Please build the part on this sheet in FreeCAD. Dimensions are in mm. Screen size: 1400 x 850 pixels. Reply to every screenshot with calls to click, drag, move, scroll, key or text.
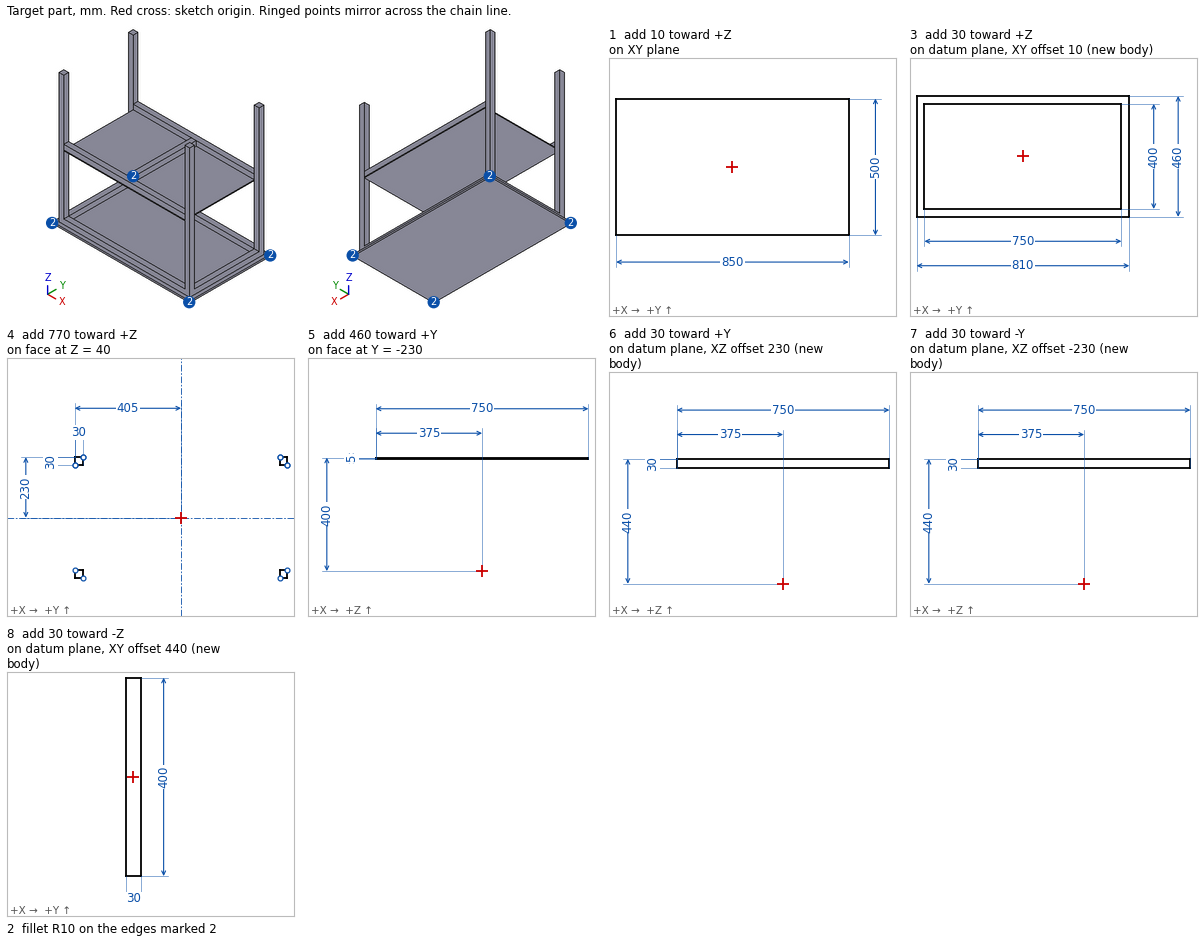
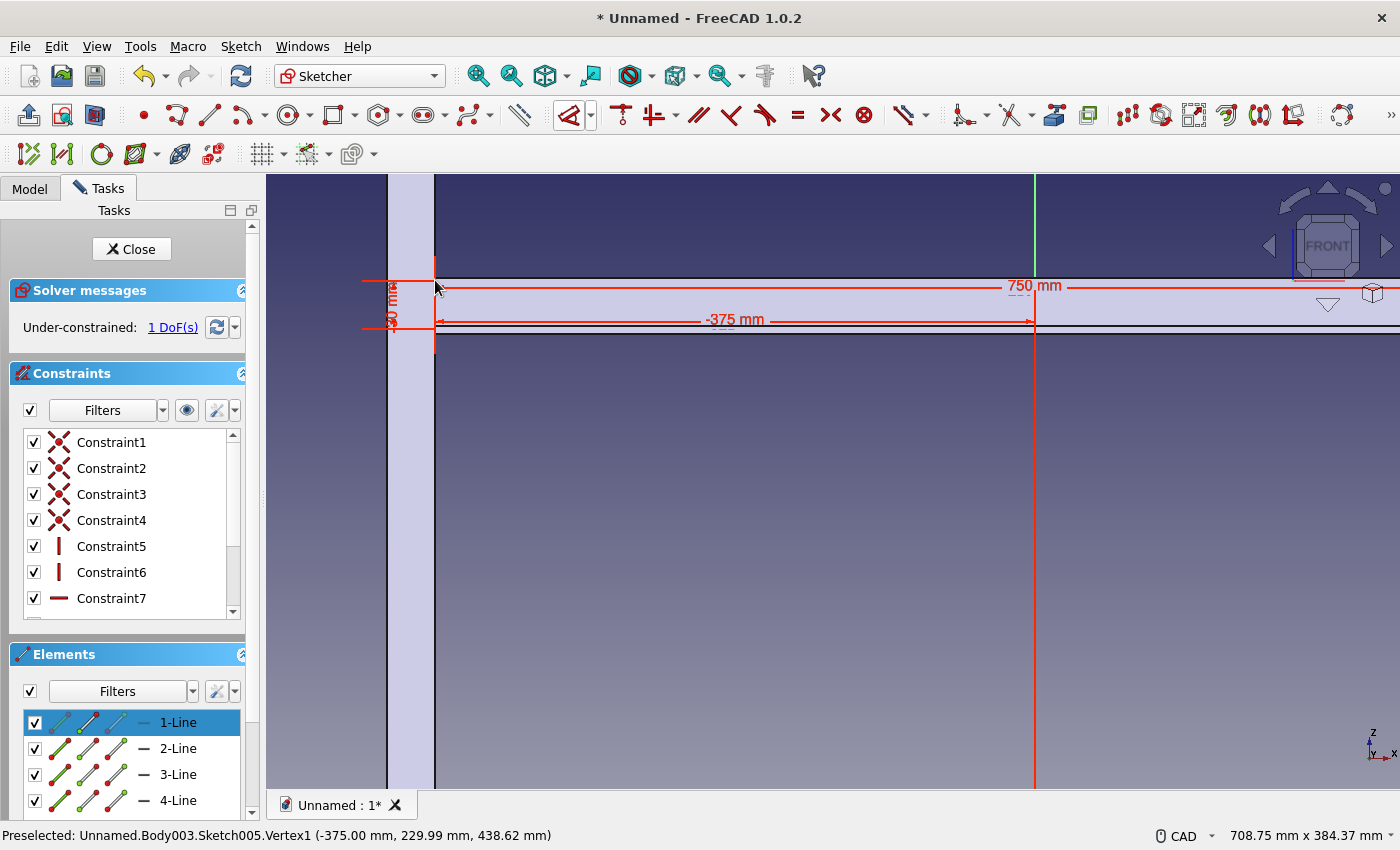
key(i)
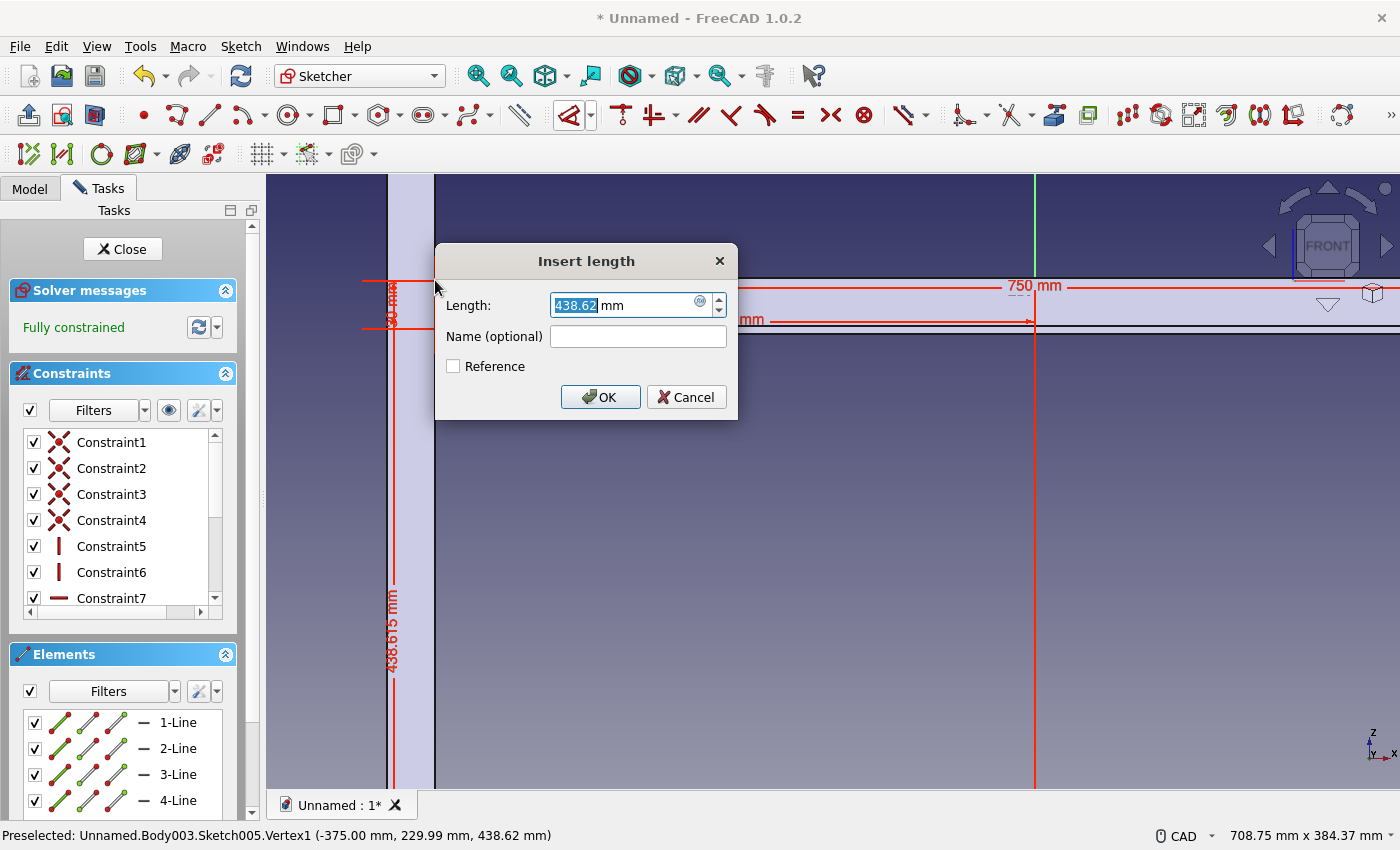
text(440)
key(Return)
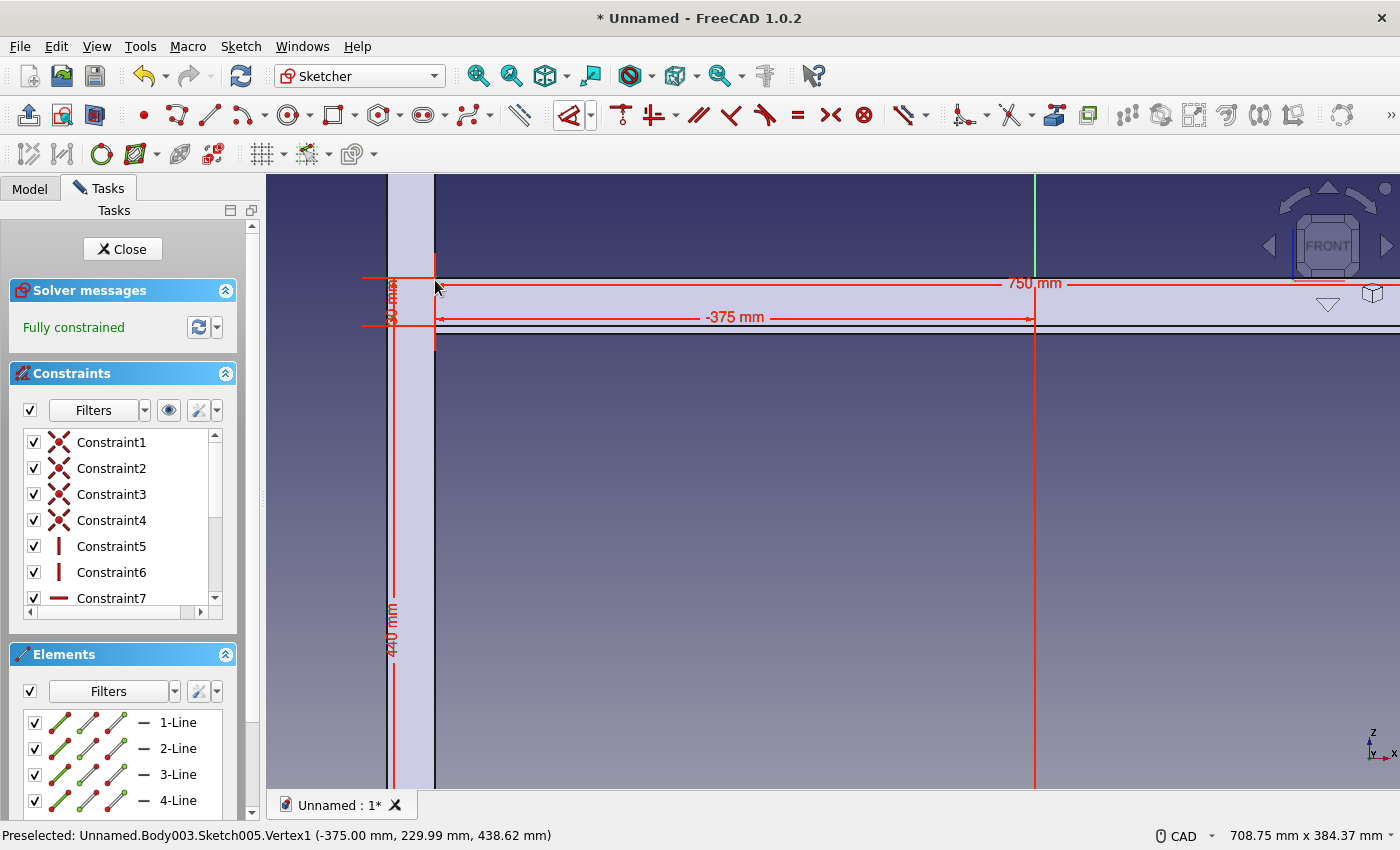
click(123, 249)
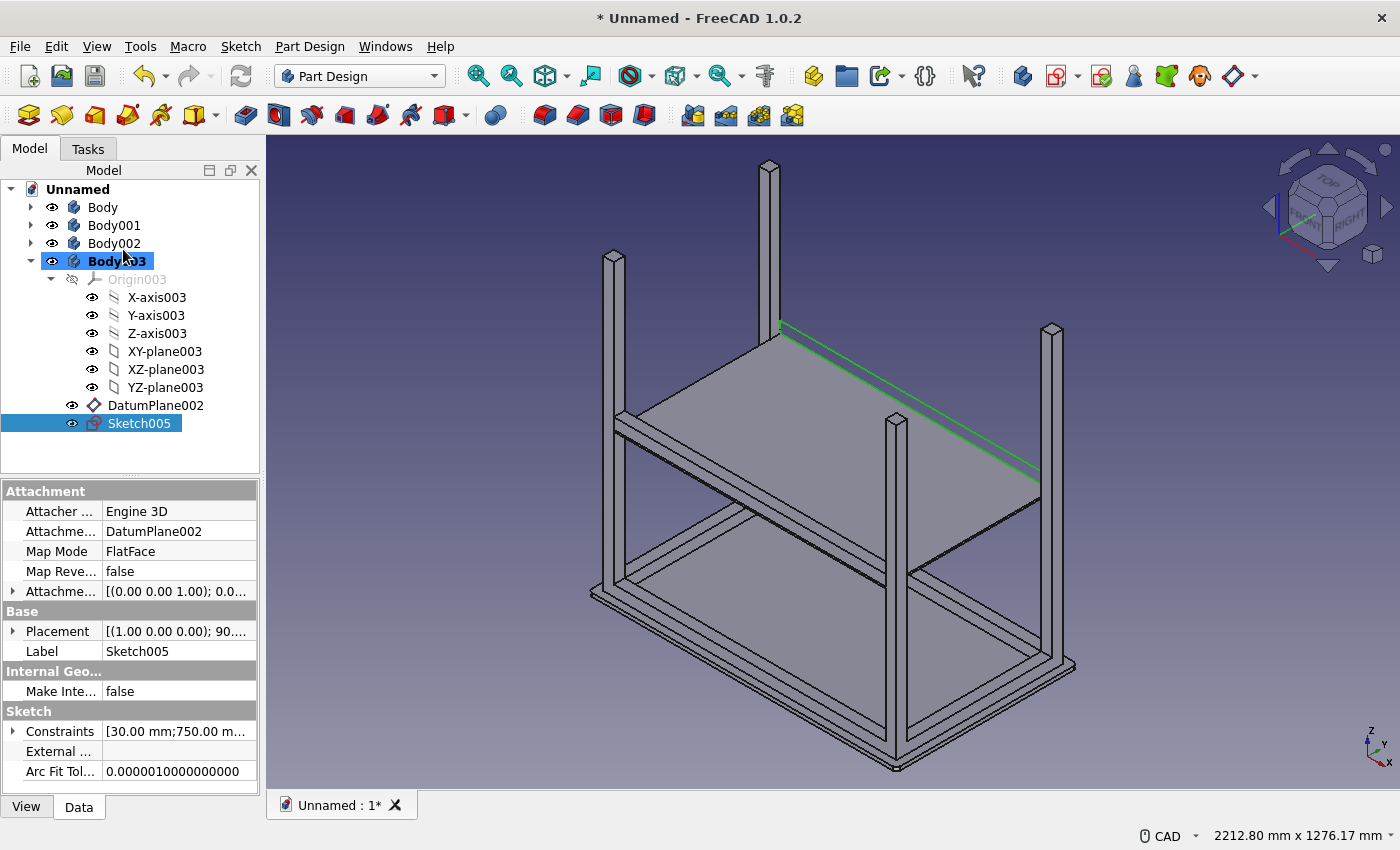
click(29, 116)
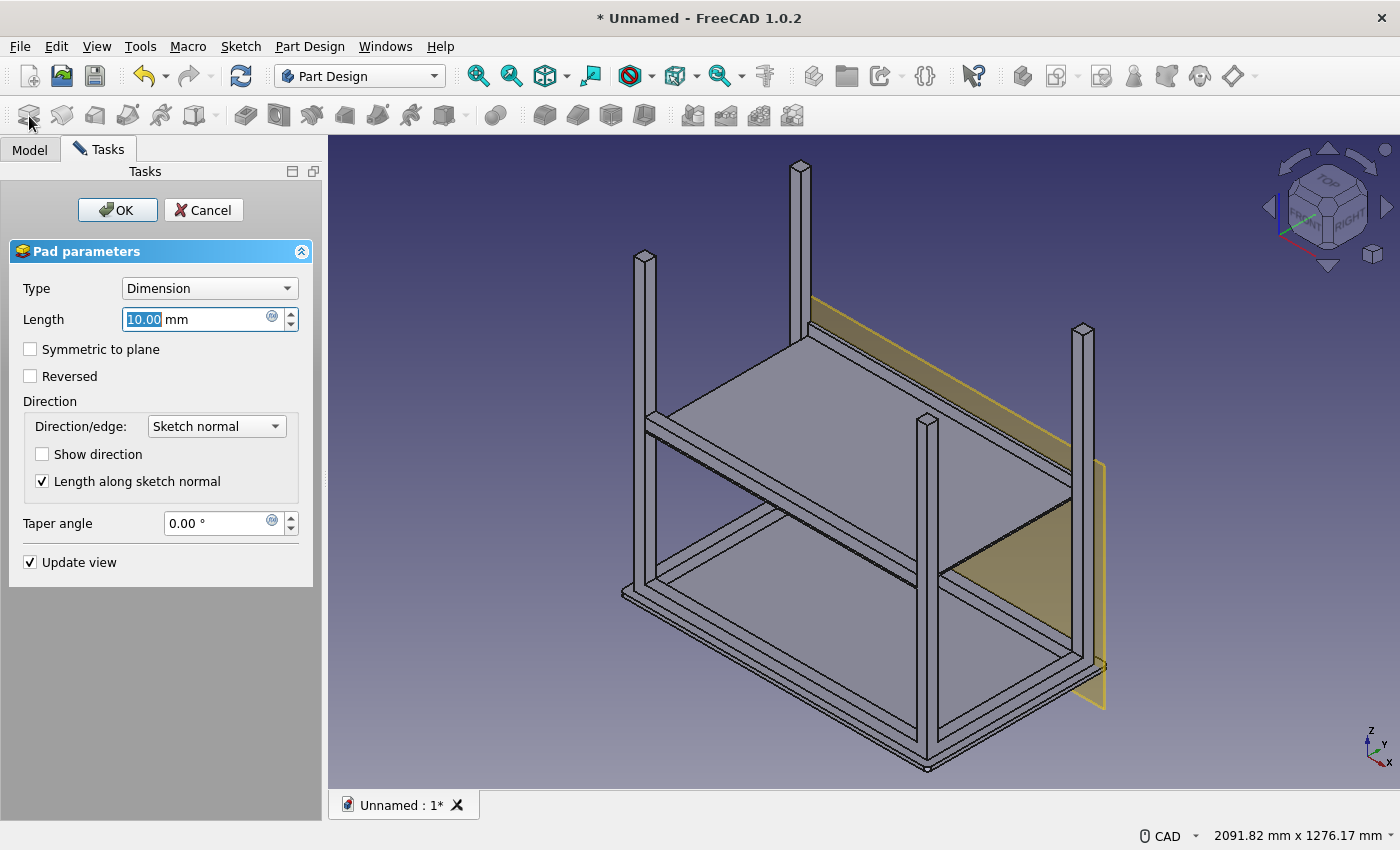
text(30)
key(Tab)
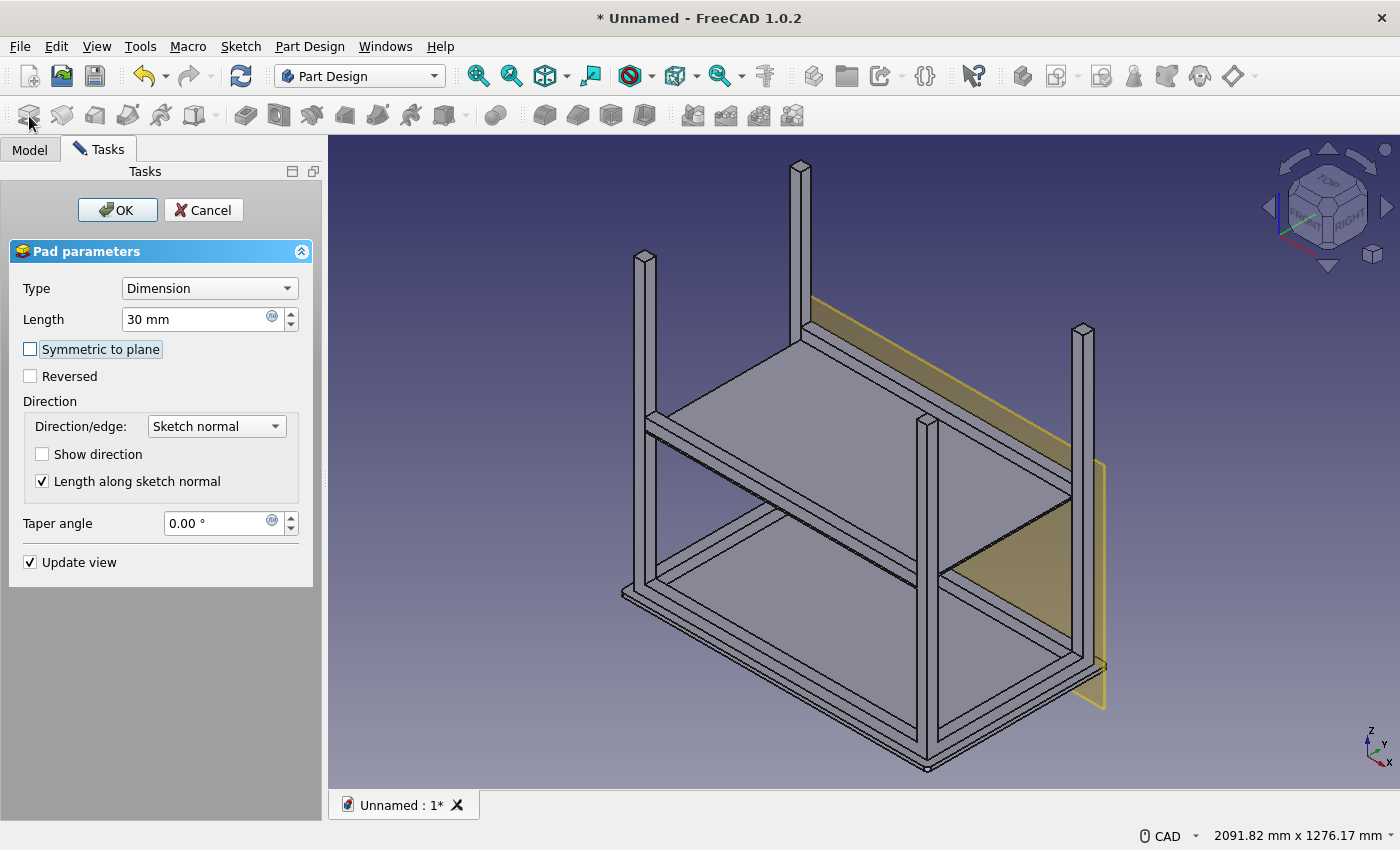
click(118, 210)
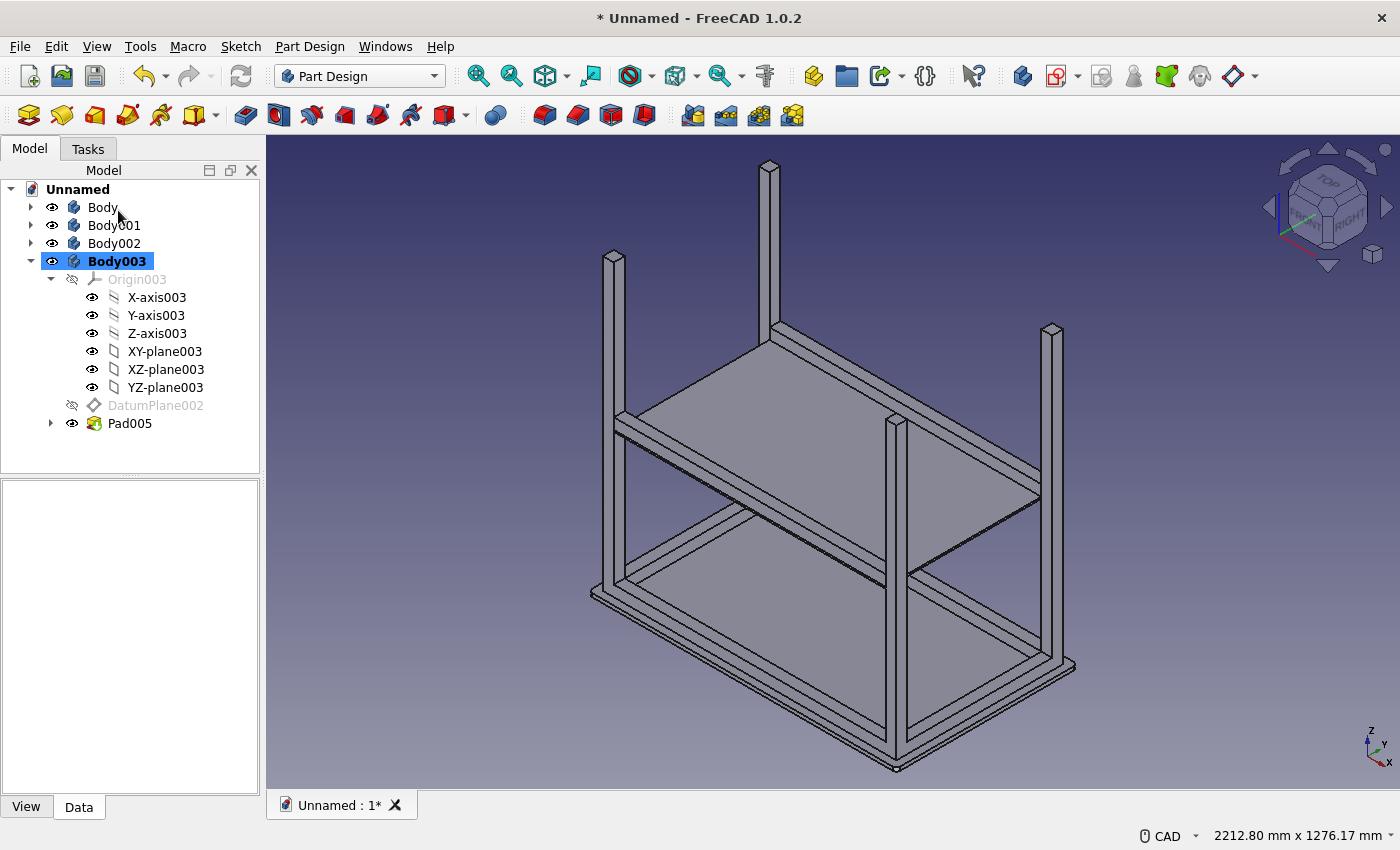
click(479, 76)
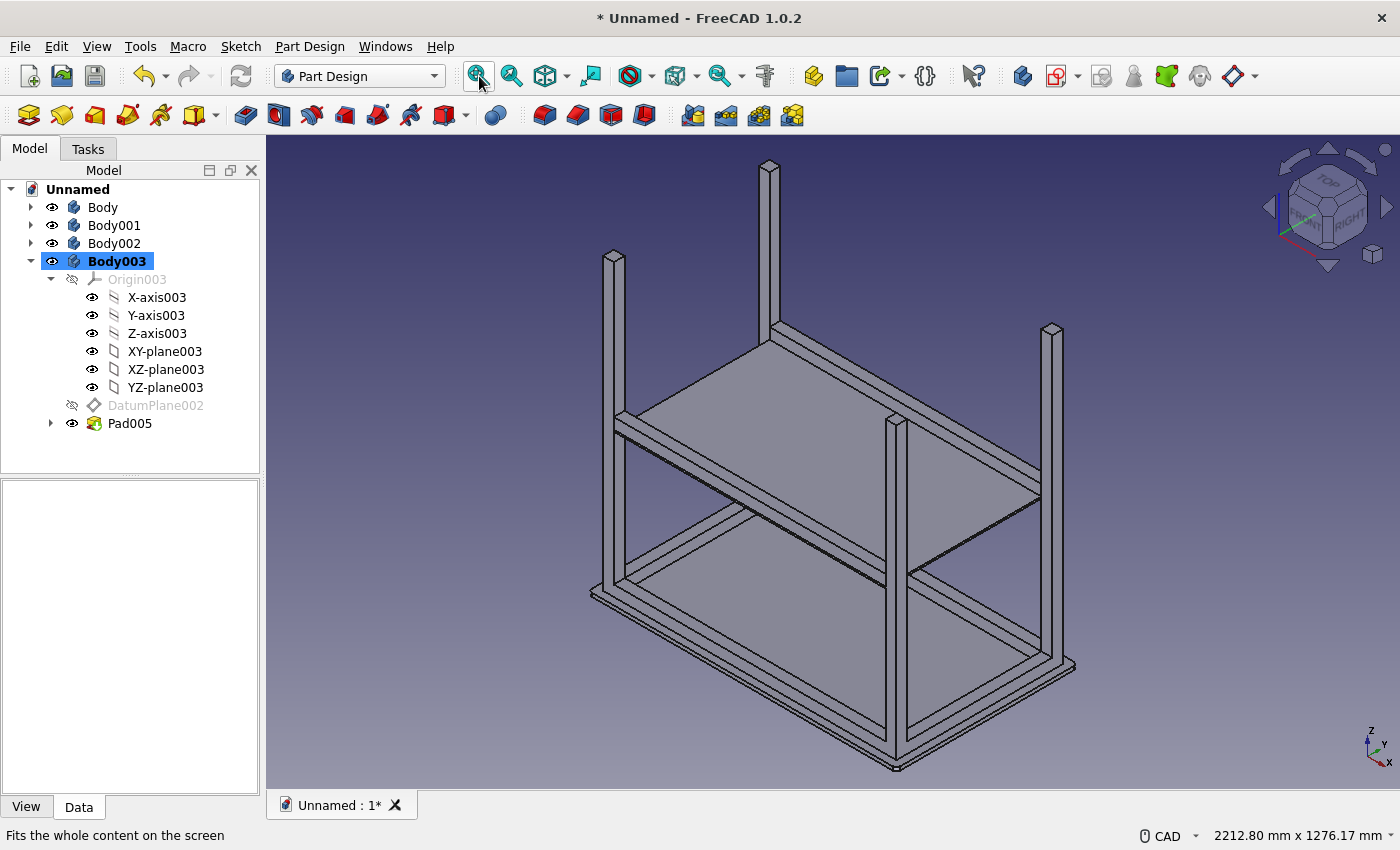
click(1023, 76)